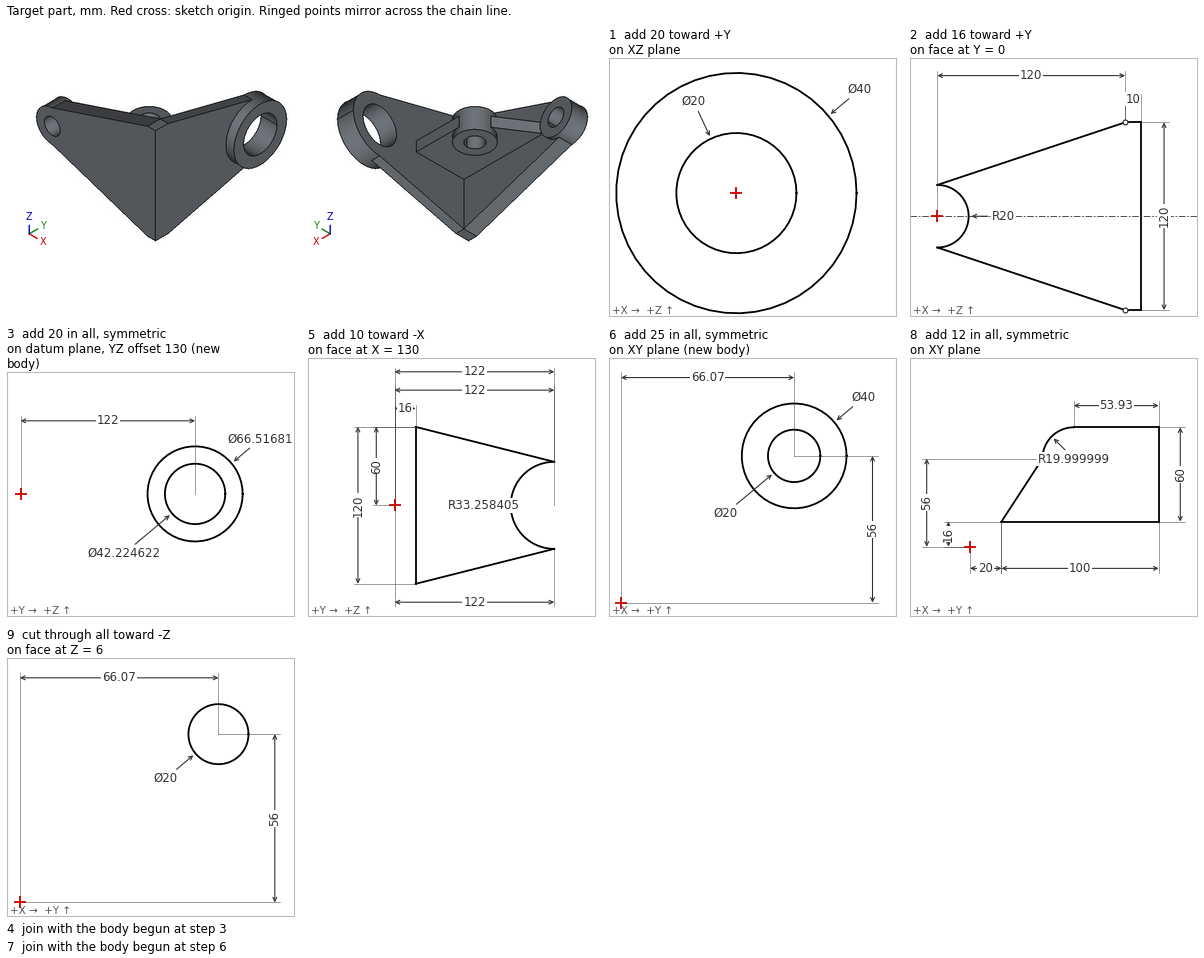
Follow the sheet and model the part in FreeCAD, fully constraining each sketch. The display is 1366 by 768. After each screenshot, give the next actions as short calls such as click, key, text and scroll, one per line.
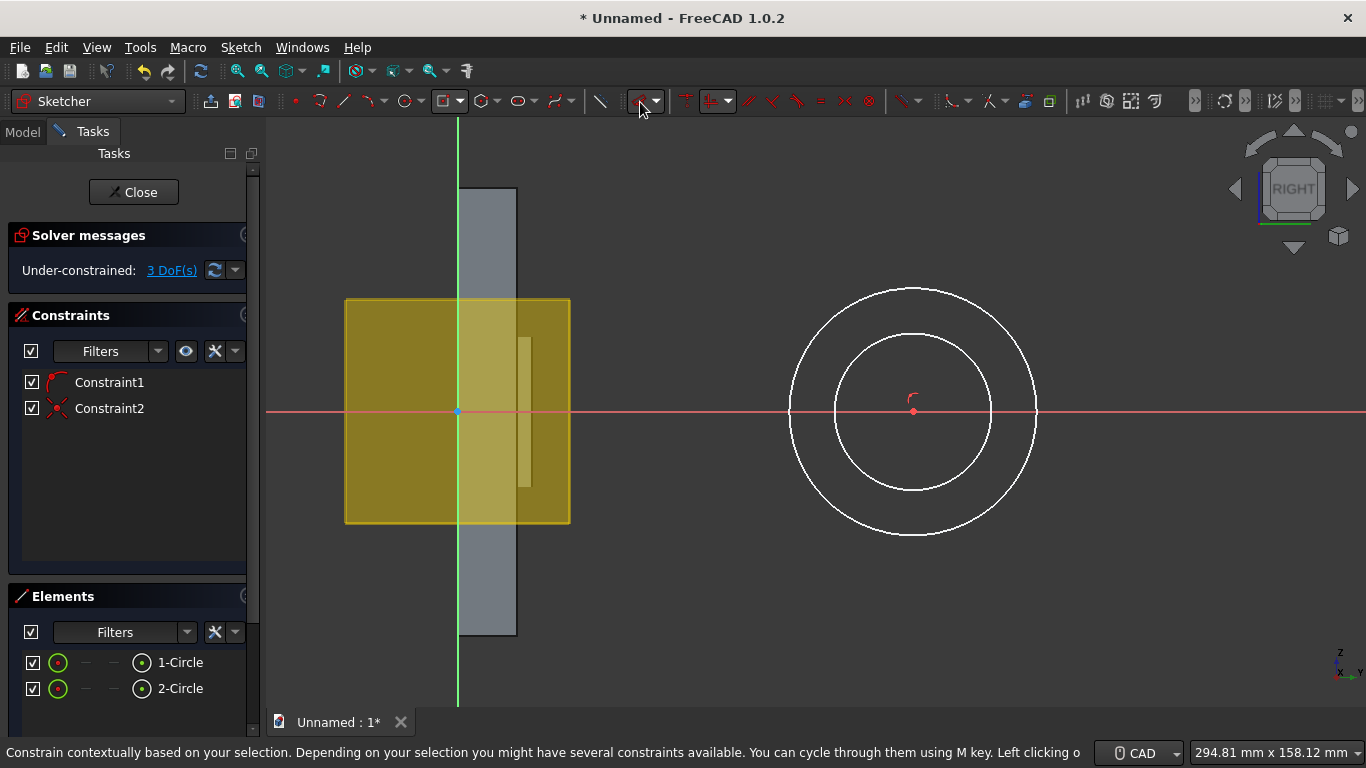
click(1000, 324)
click(1023, 301)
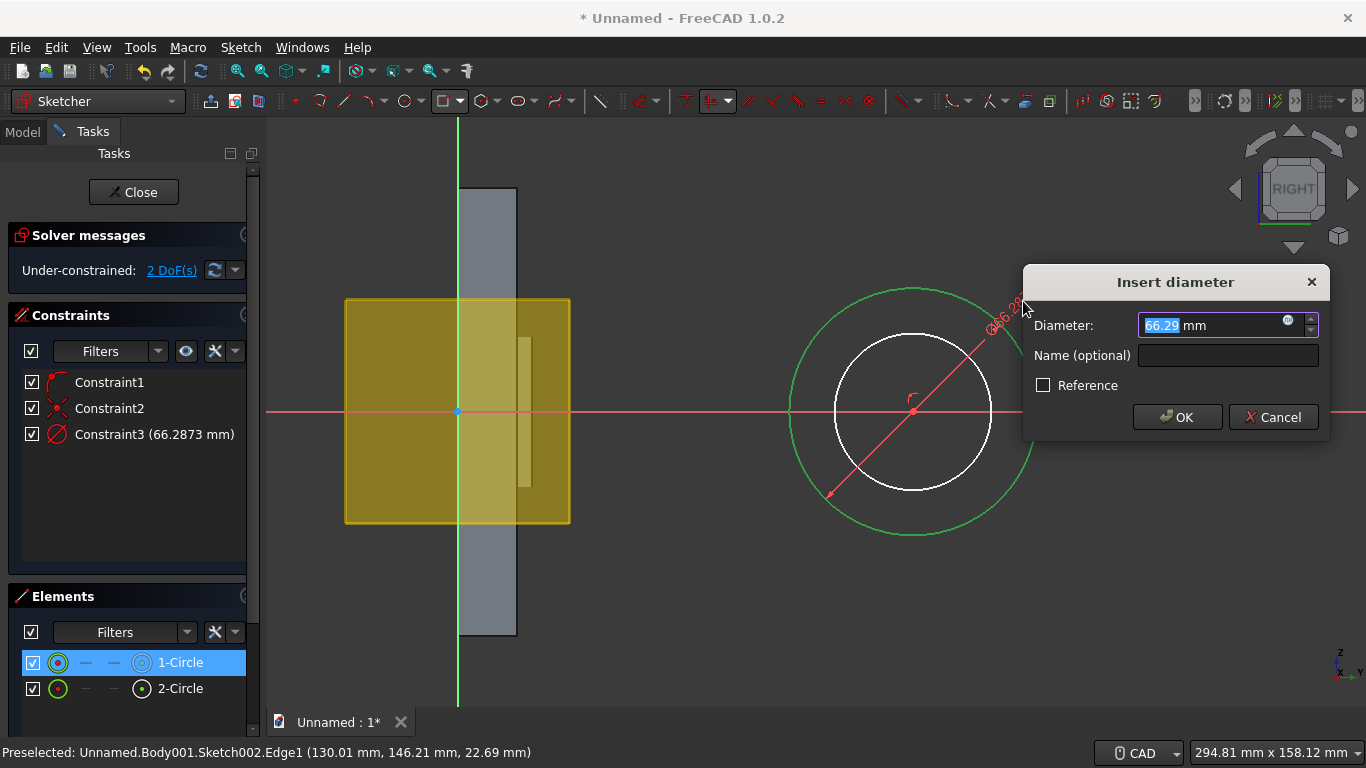
text(66.51681)
key(Return)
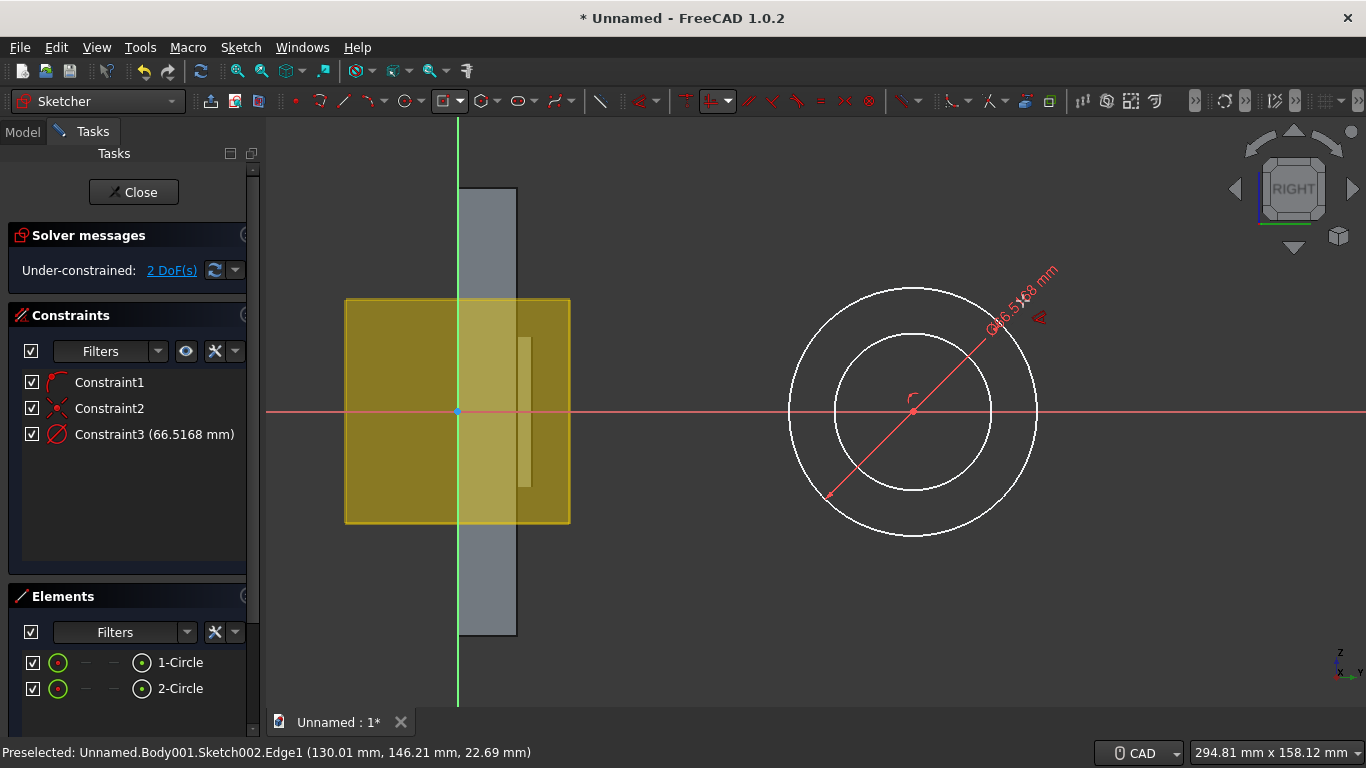
click(968, 356)
click(990, 333)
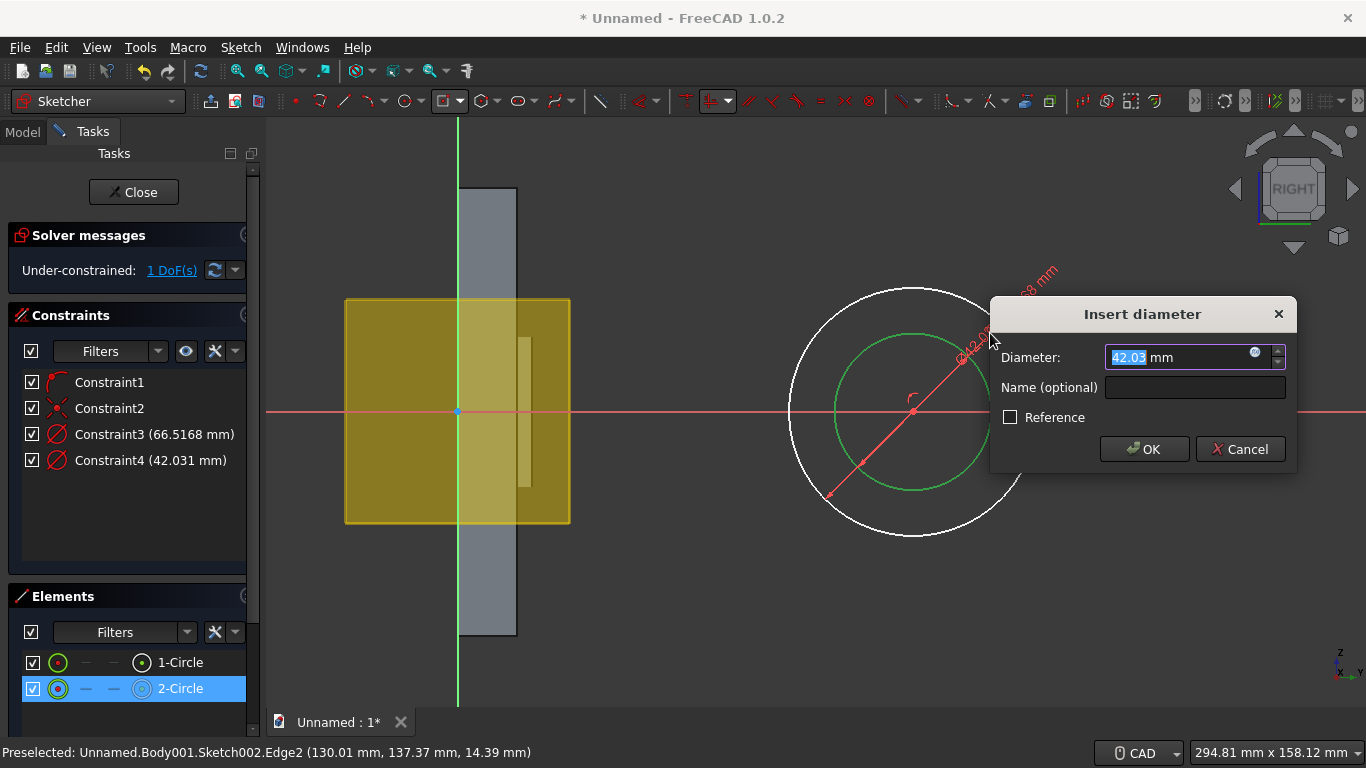
text(42.224622)
key(Return)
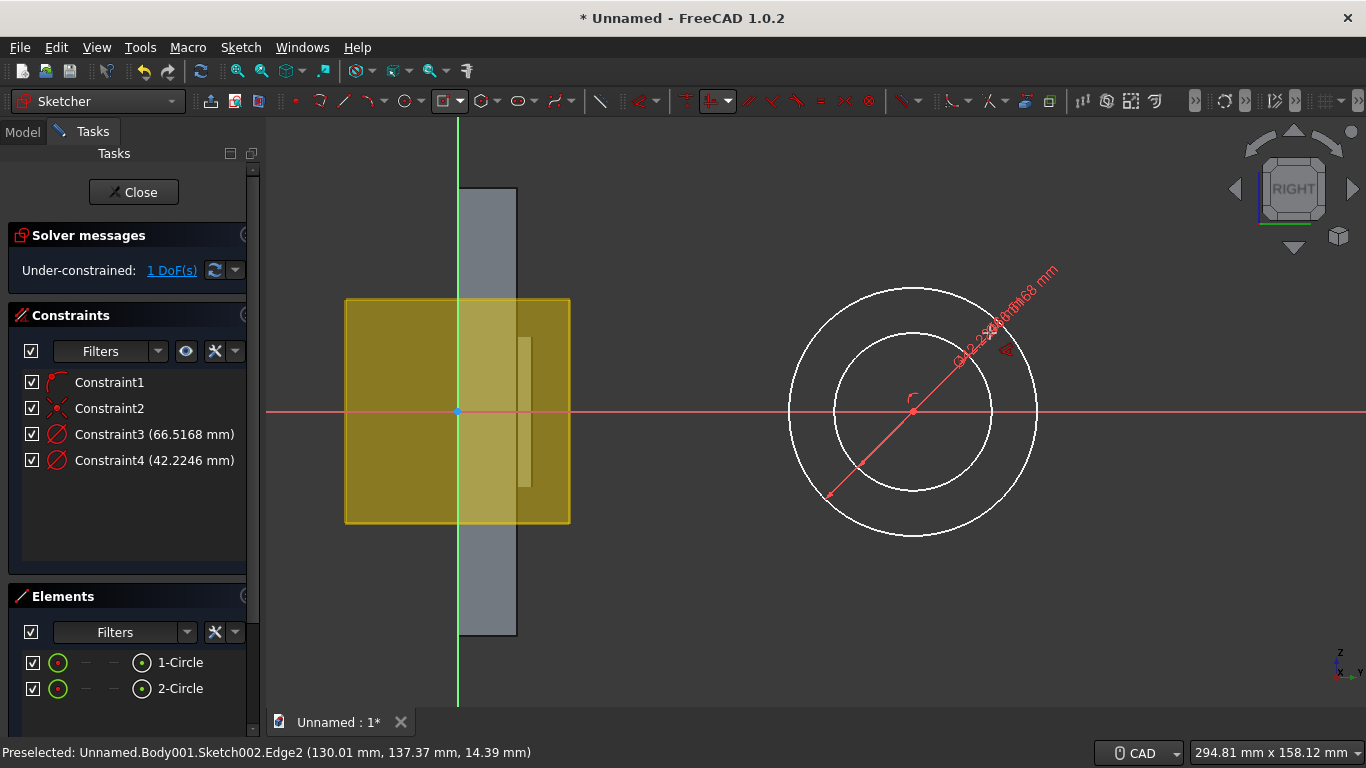
click(913, 412)
click(685, 446)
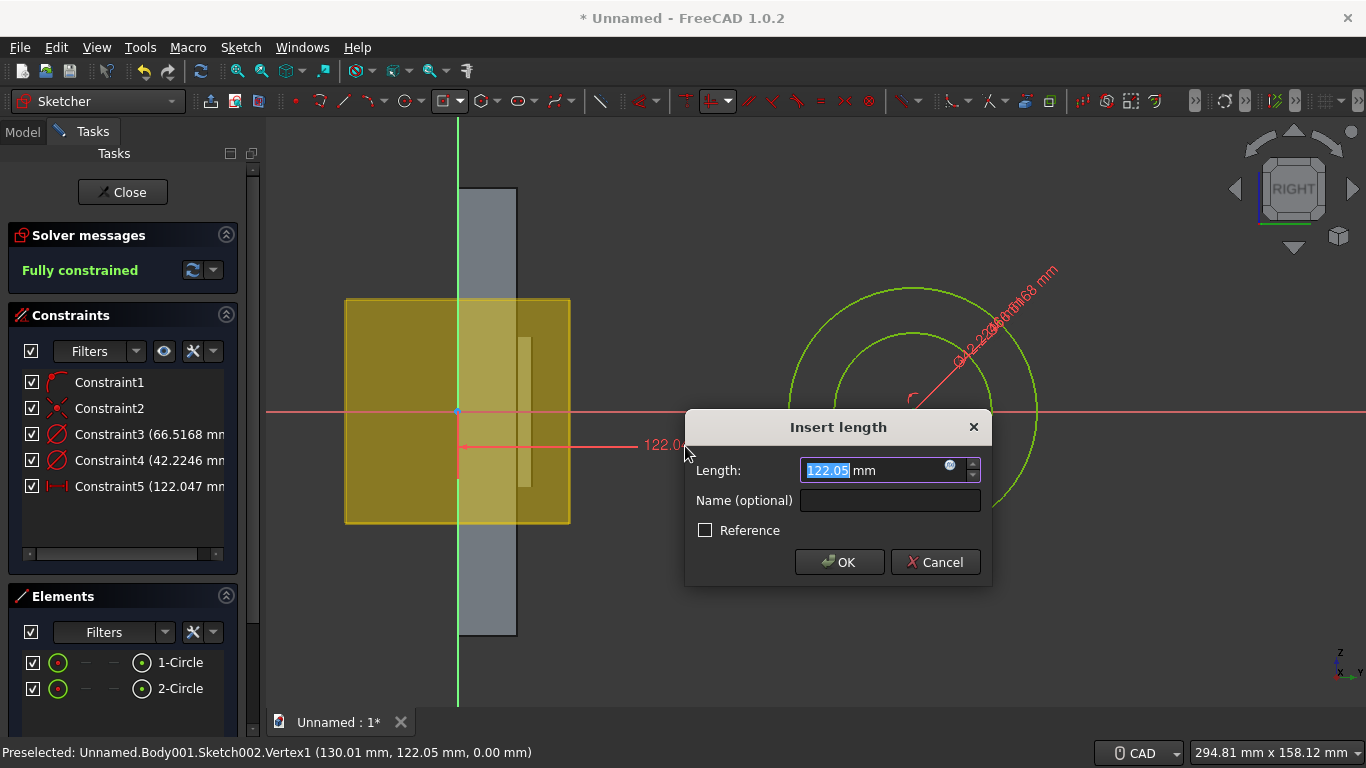
text(122)
key(Return)
key(Escape)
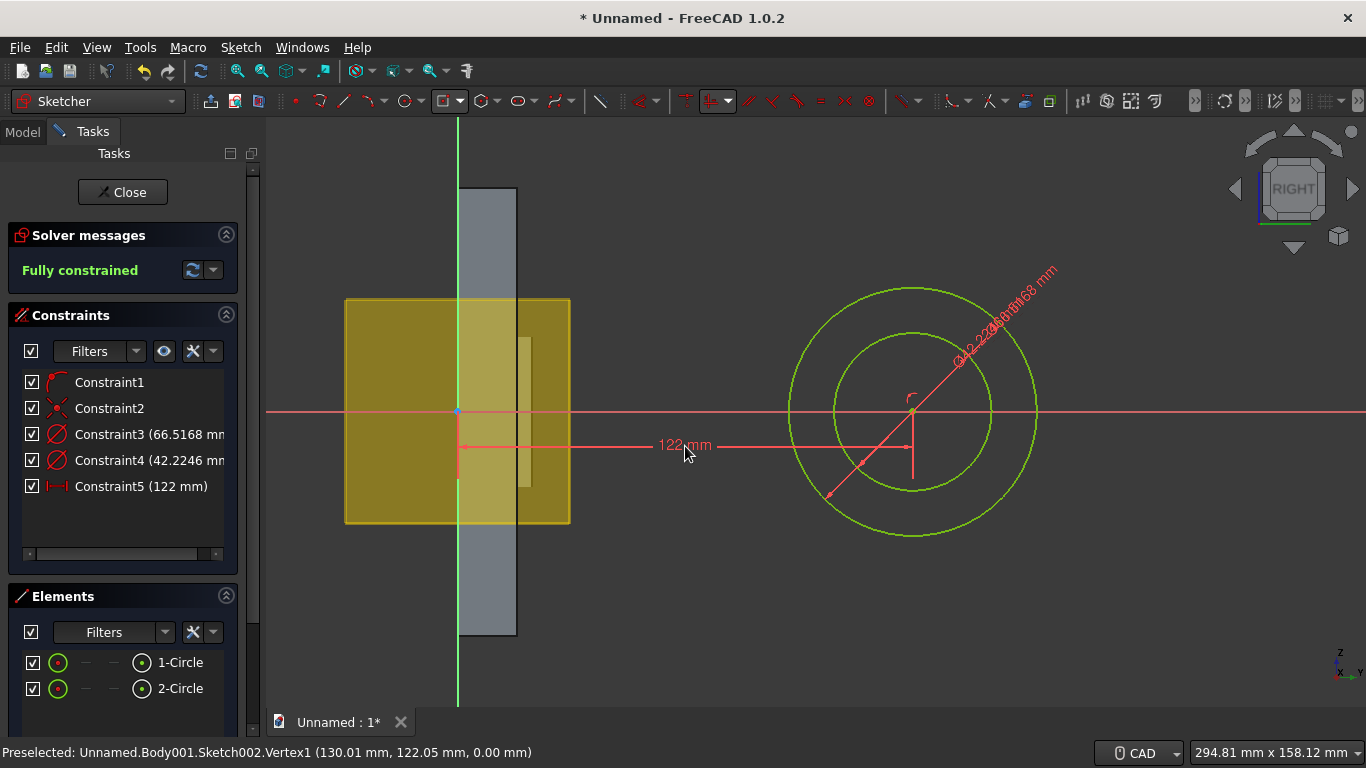
click(123, 192)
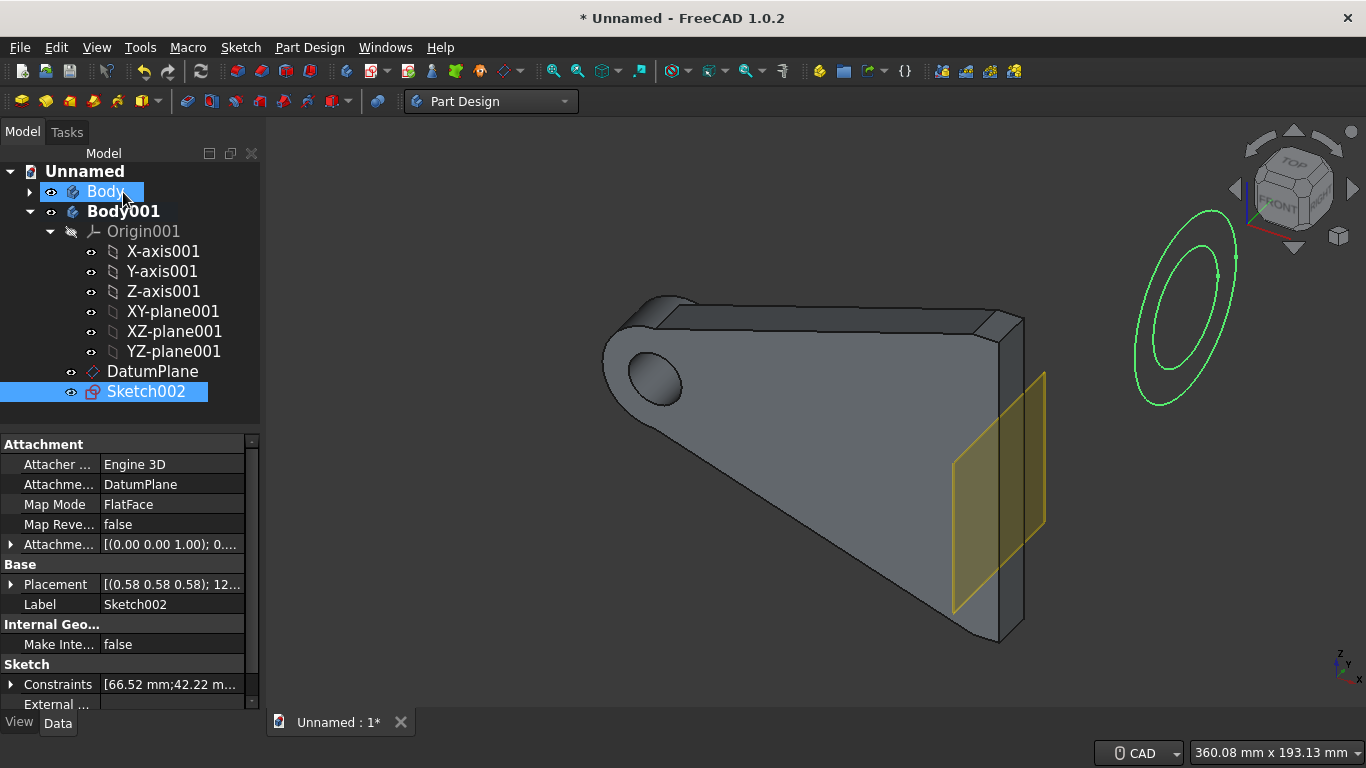
click(22, 102)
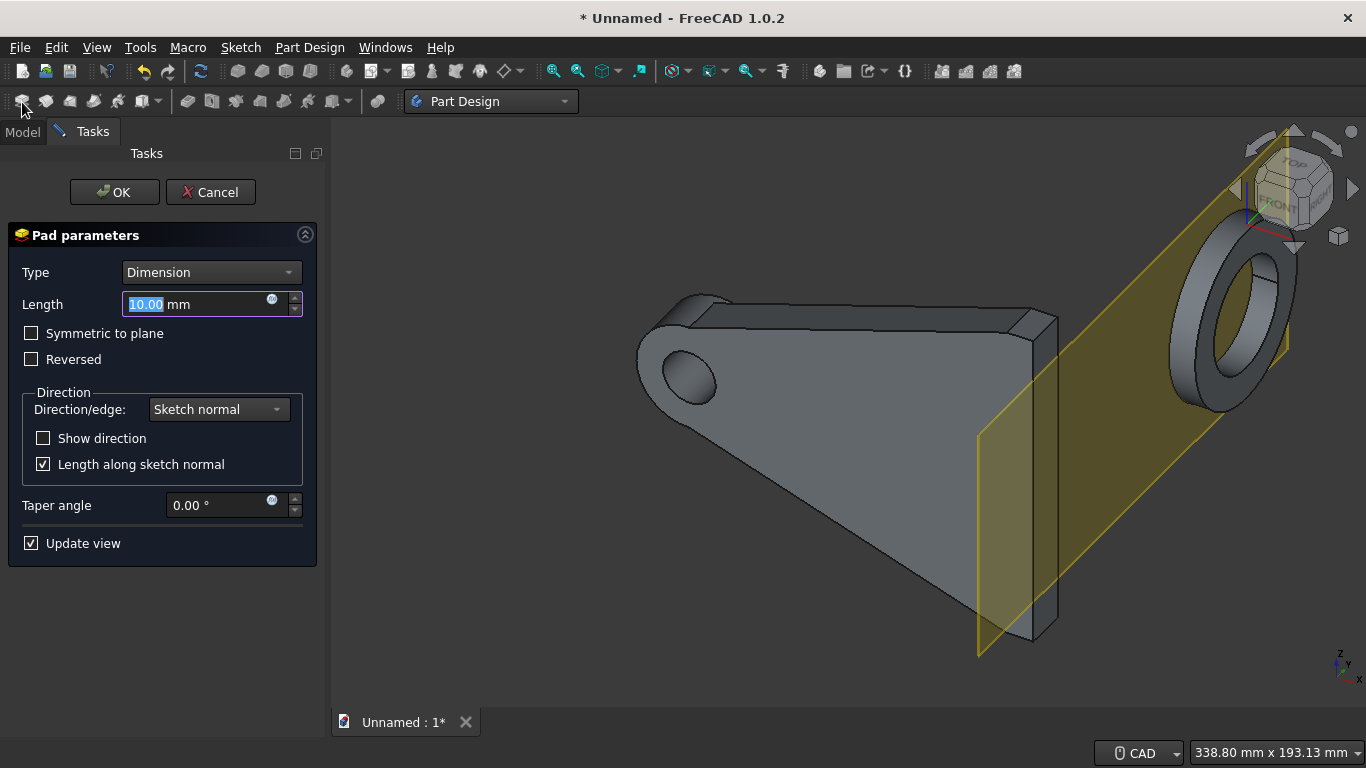
text(20)
key(Tab)